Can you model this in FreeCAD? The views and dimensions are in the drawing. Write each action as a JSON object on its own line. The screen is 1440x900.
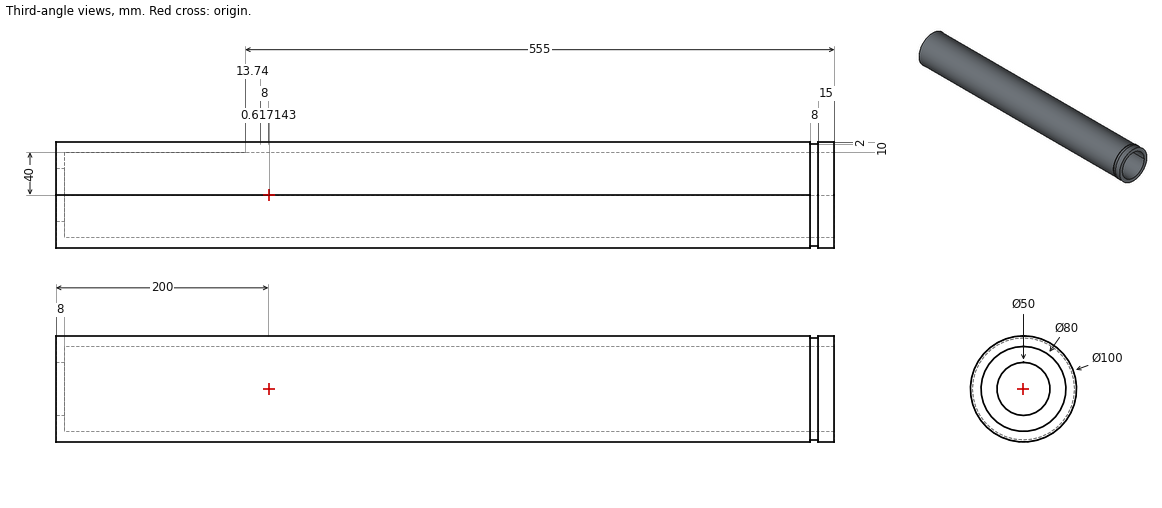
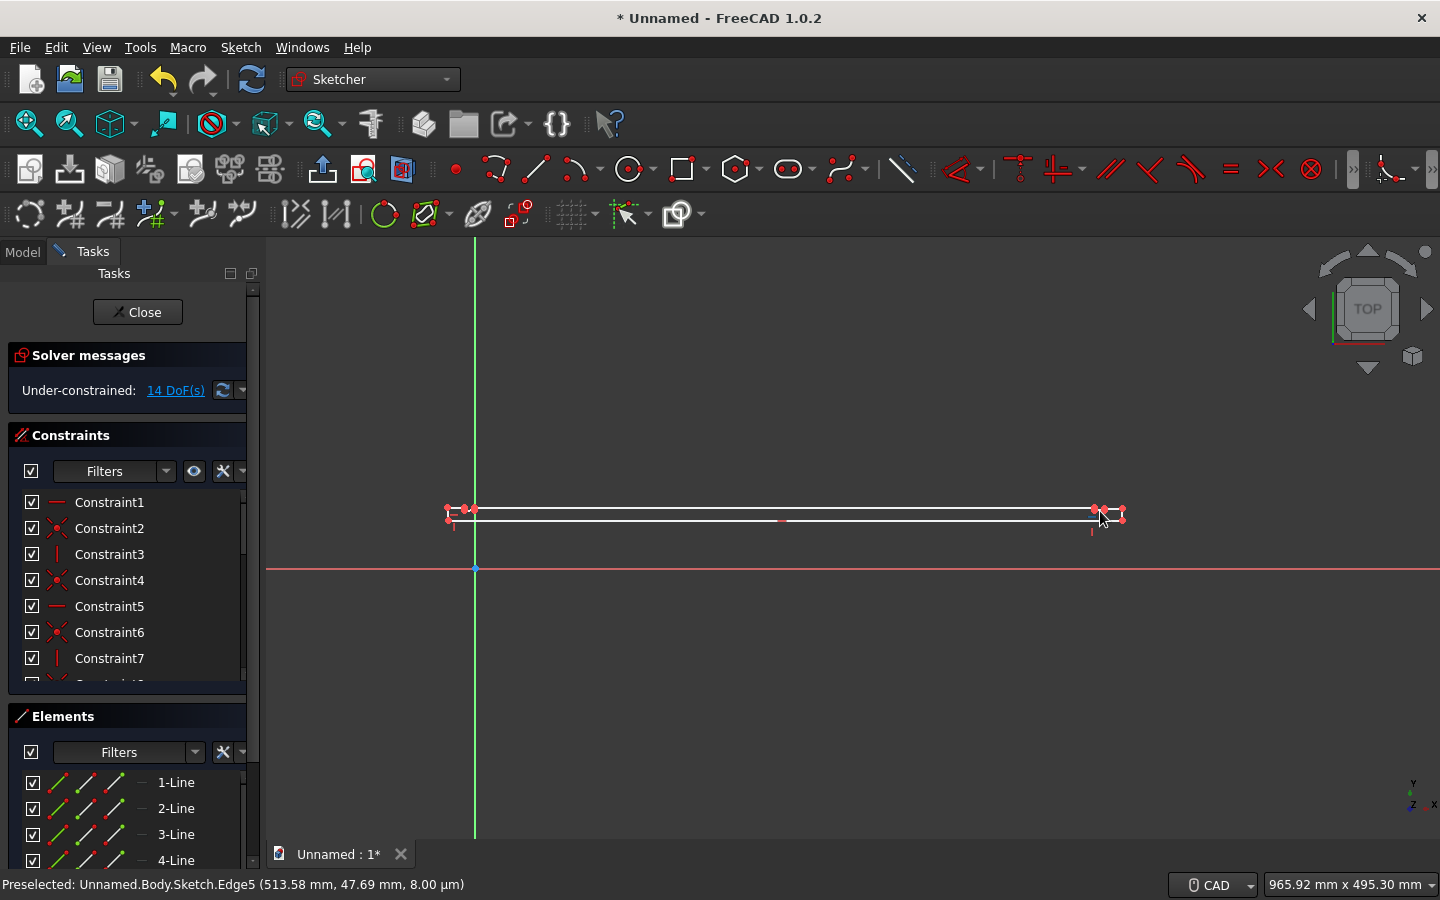
{"action": "scroll", "coordinate": [471, 510], "scroll_direction": "up", "scroll_amount": 8}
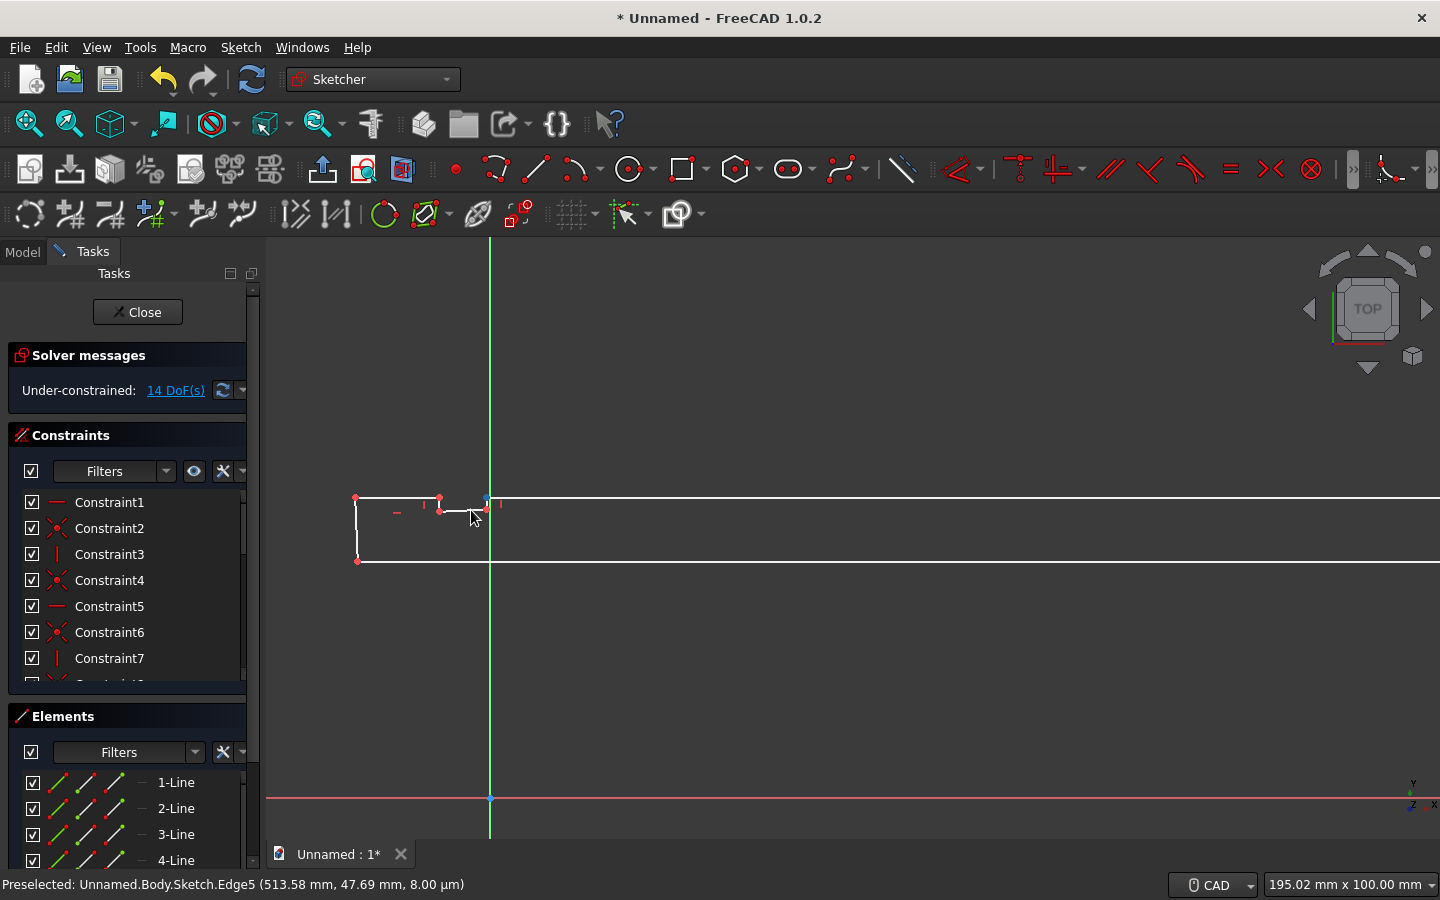
{"action": "left_click", "coordinate": [472, 510]}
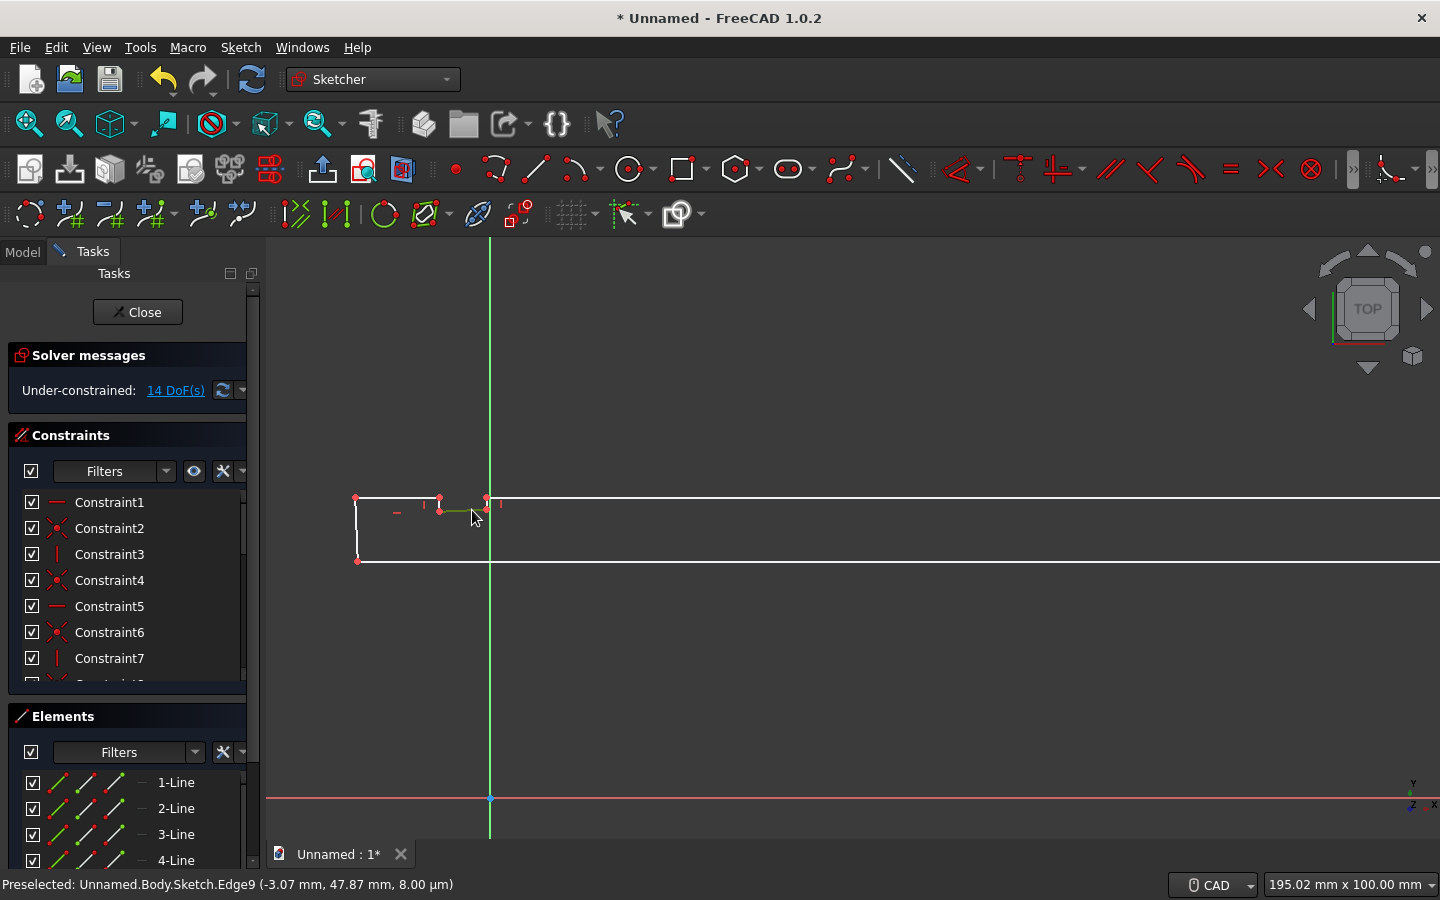
{"action": "key", "text": "h"}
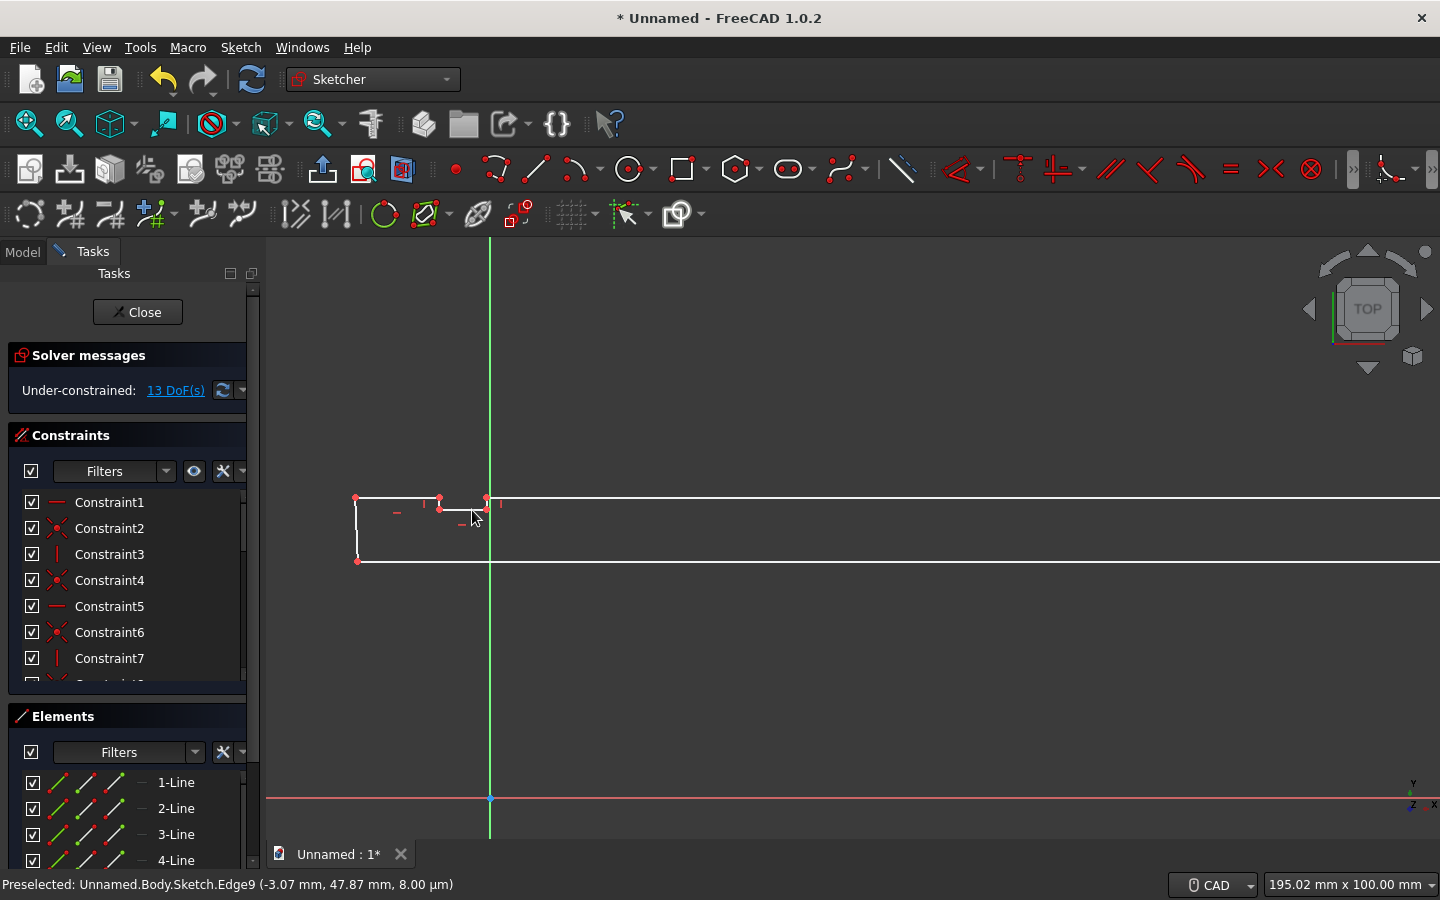
{"action": "left_click", "coordinate": [356, 517]}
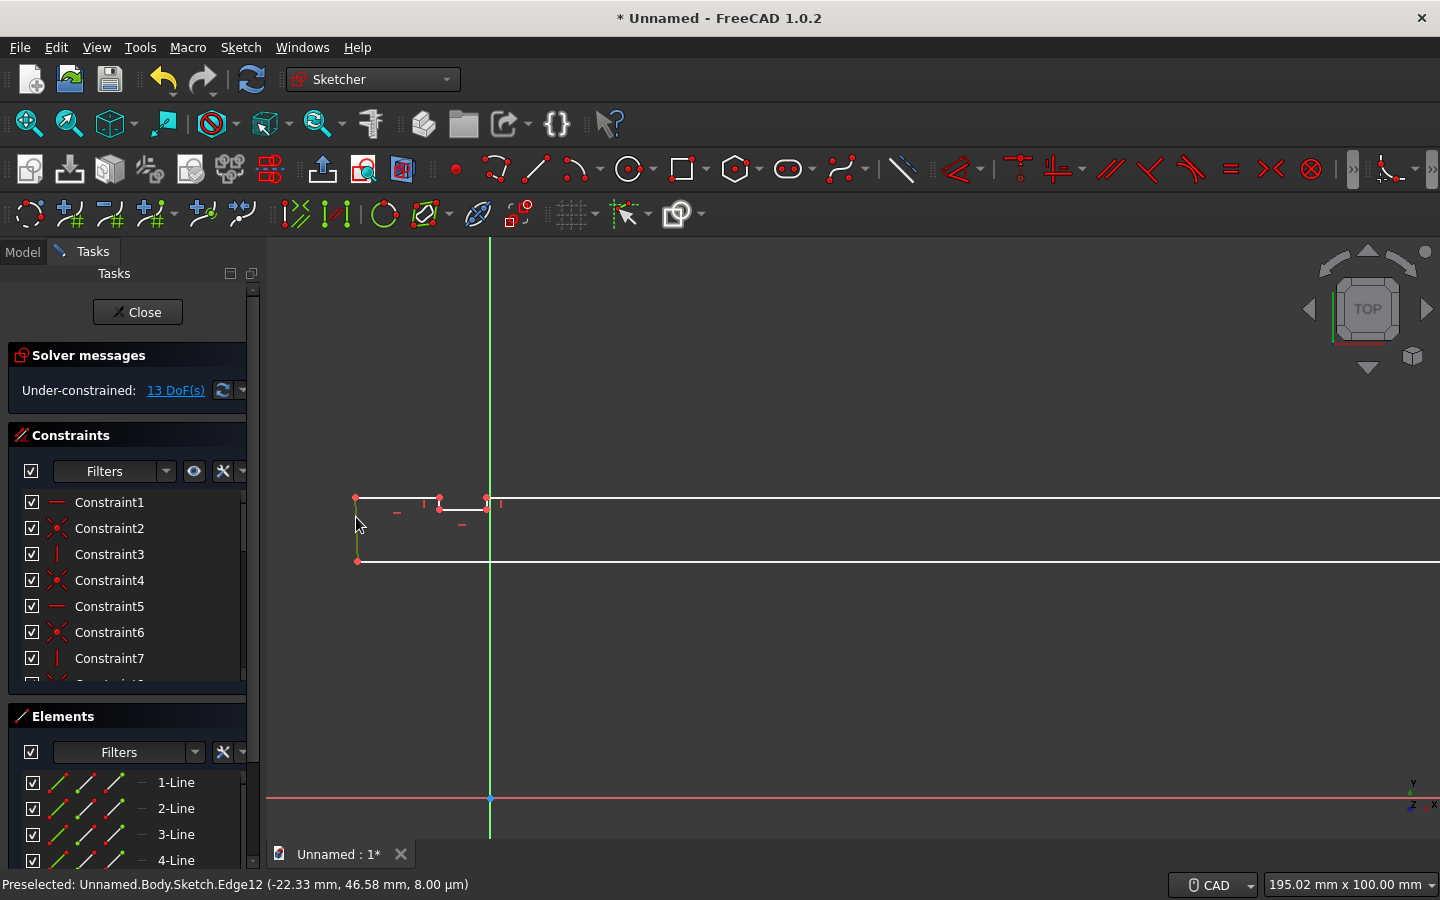
{"action": "key", "text": "v"}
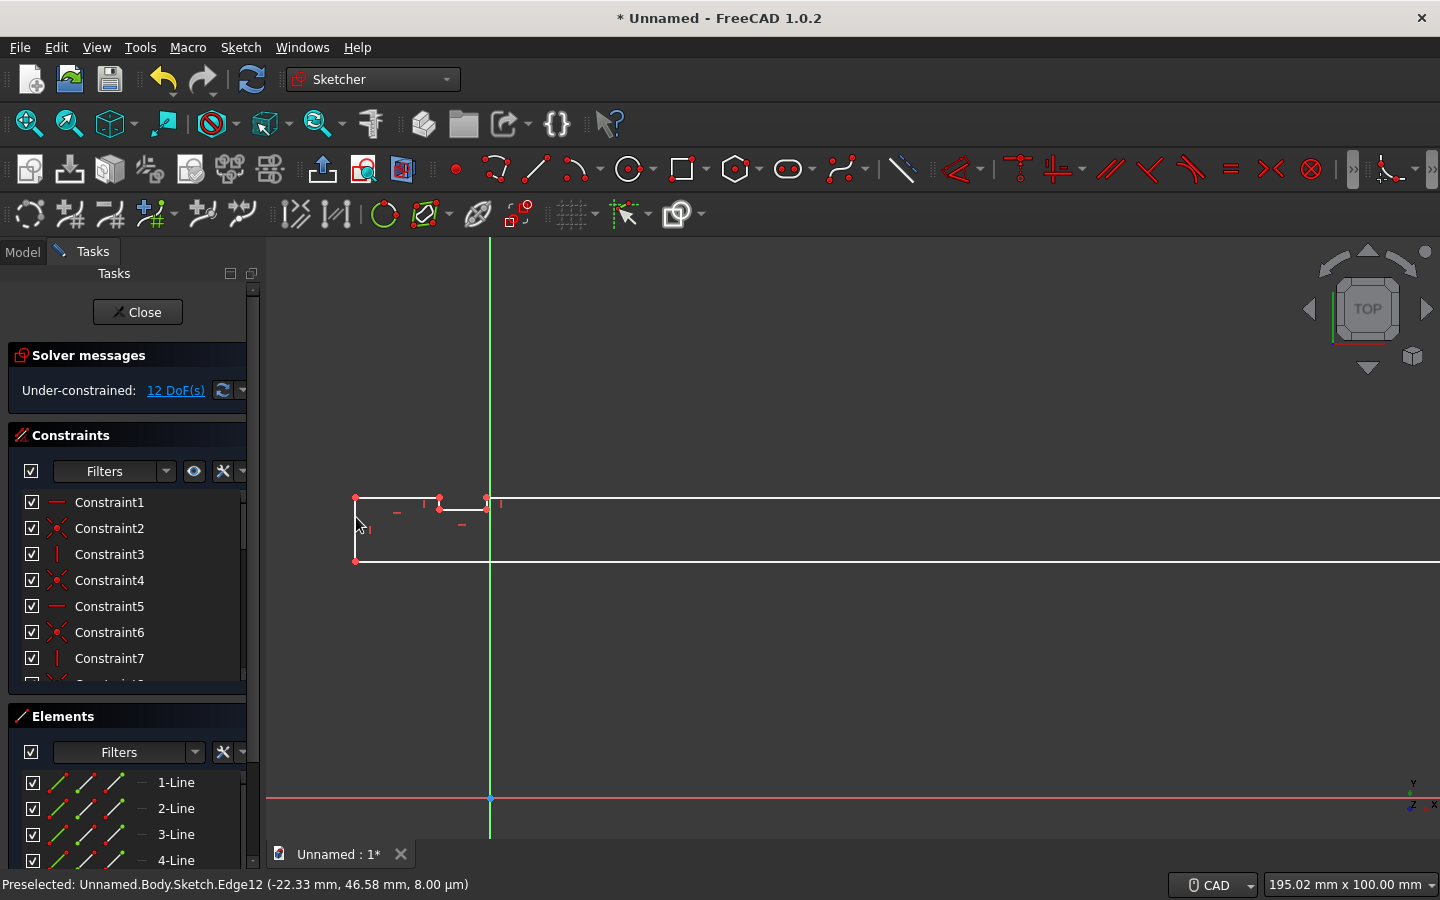
{"action": "scroll", "coordinate": [470, 510], "scroll_direction": "down", "scroll_amount": 8}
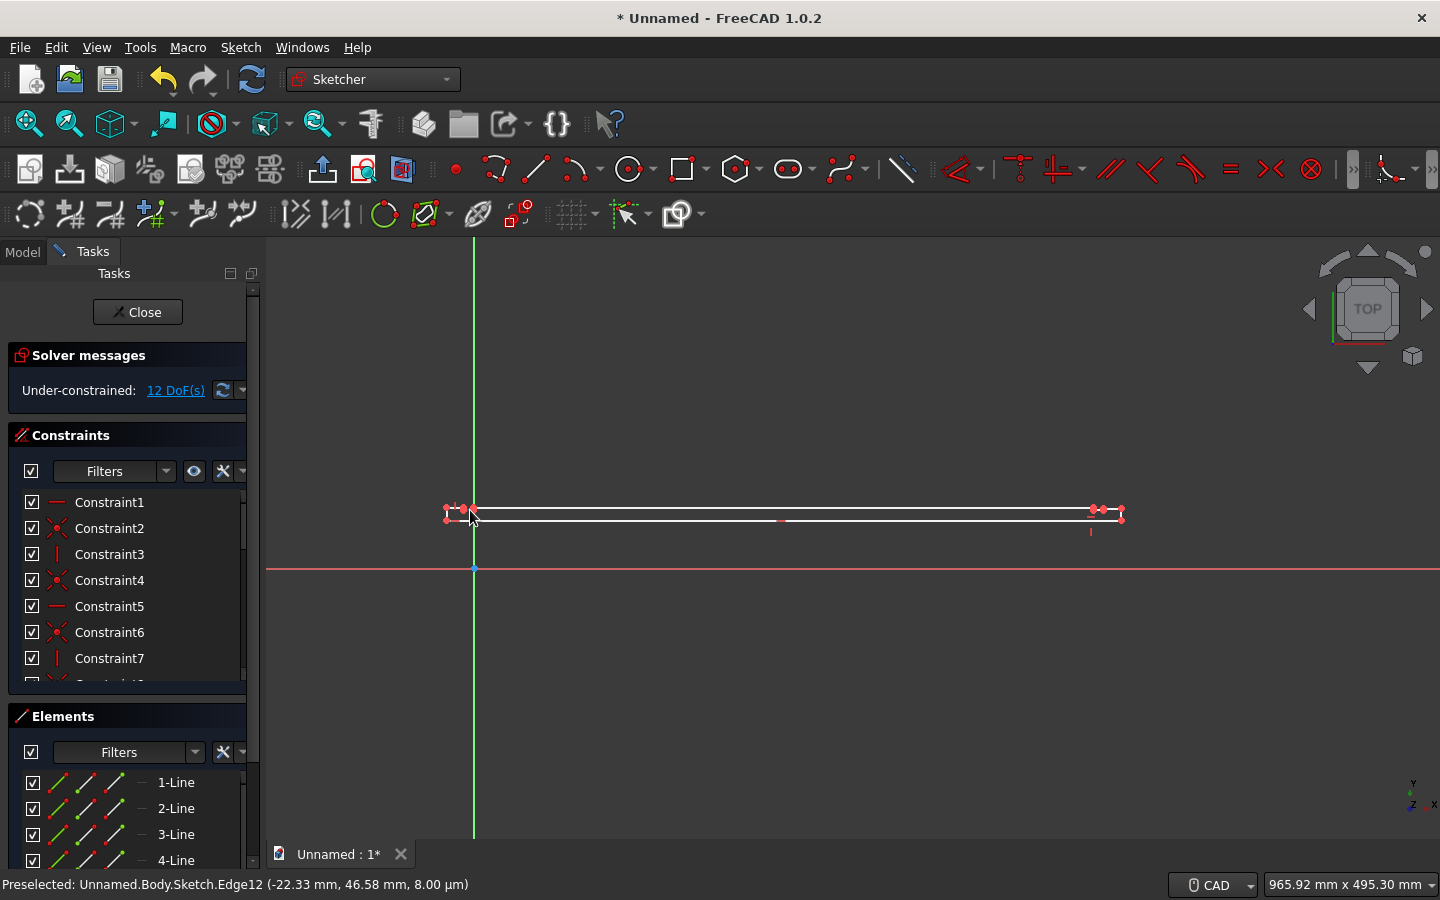
{"action": "scroll", "coordinate": [1104, 509], "scroll_direction": "up", "scroll_amount": 14}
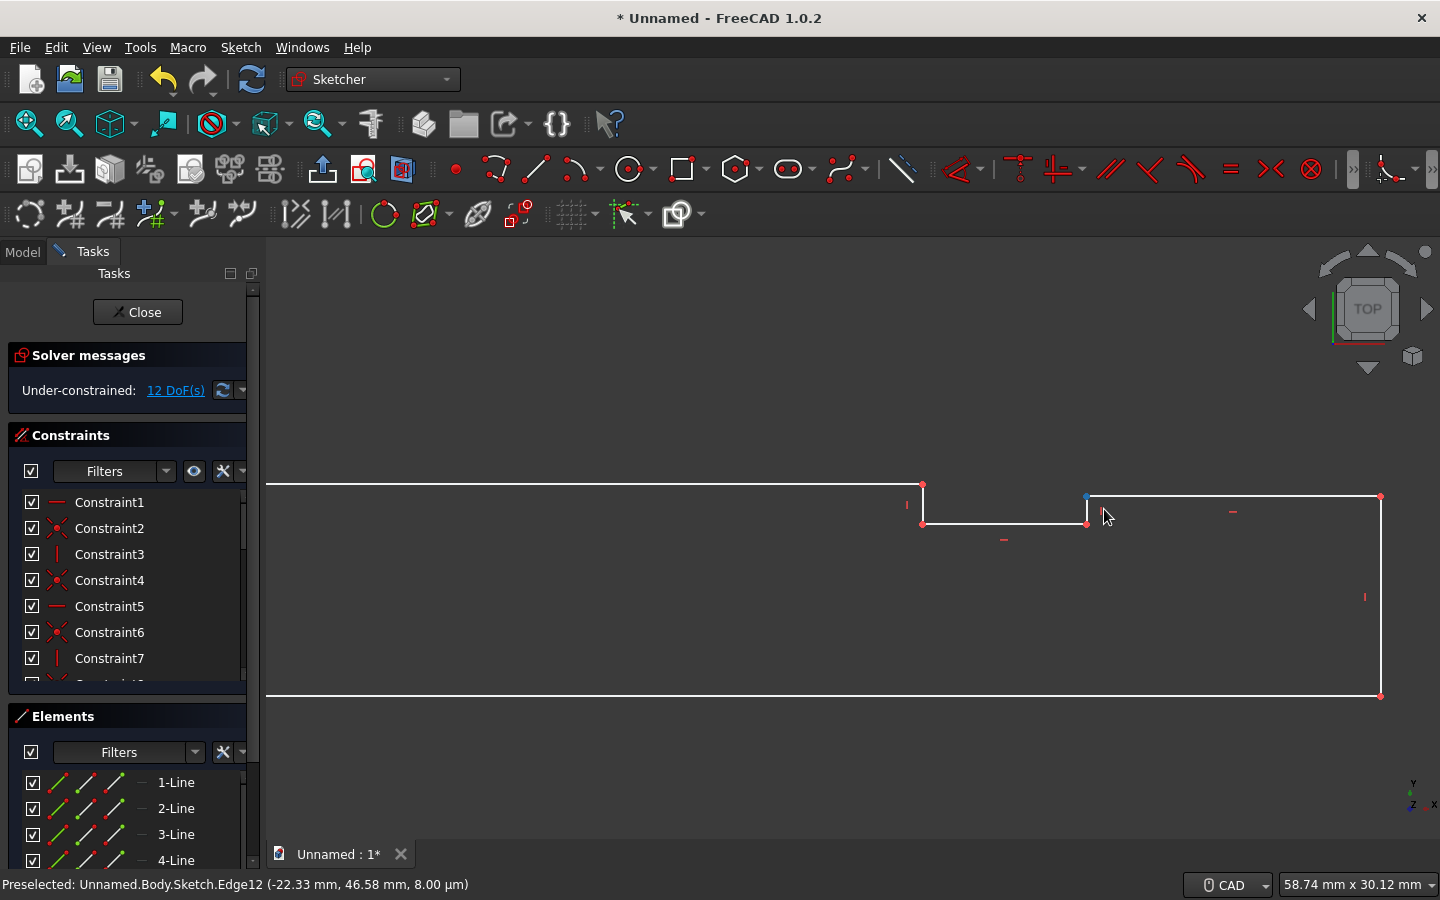
{"action": "left_click", "coordinate": [1087, 510]}